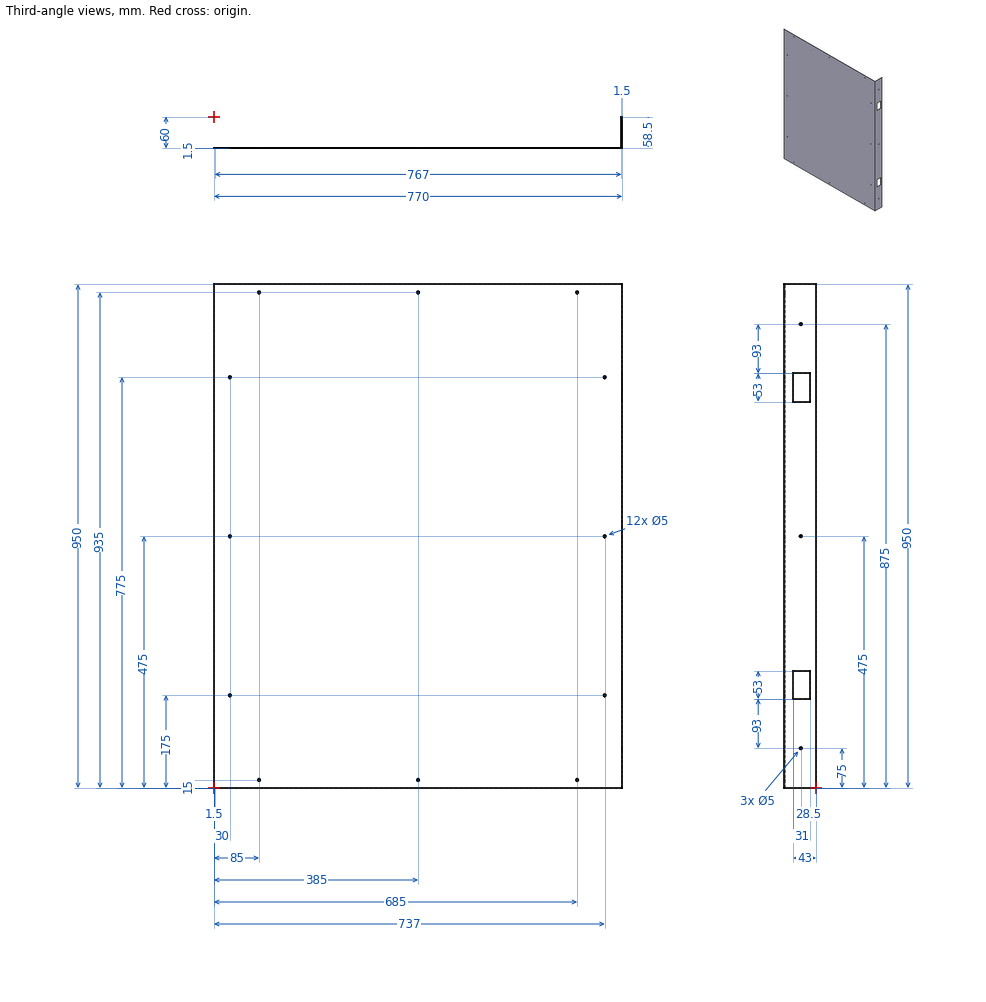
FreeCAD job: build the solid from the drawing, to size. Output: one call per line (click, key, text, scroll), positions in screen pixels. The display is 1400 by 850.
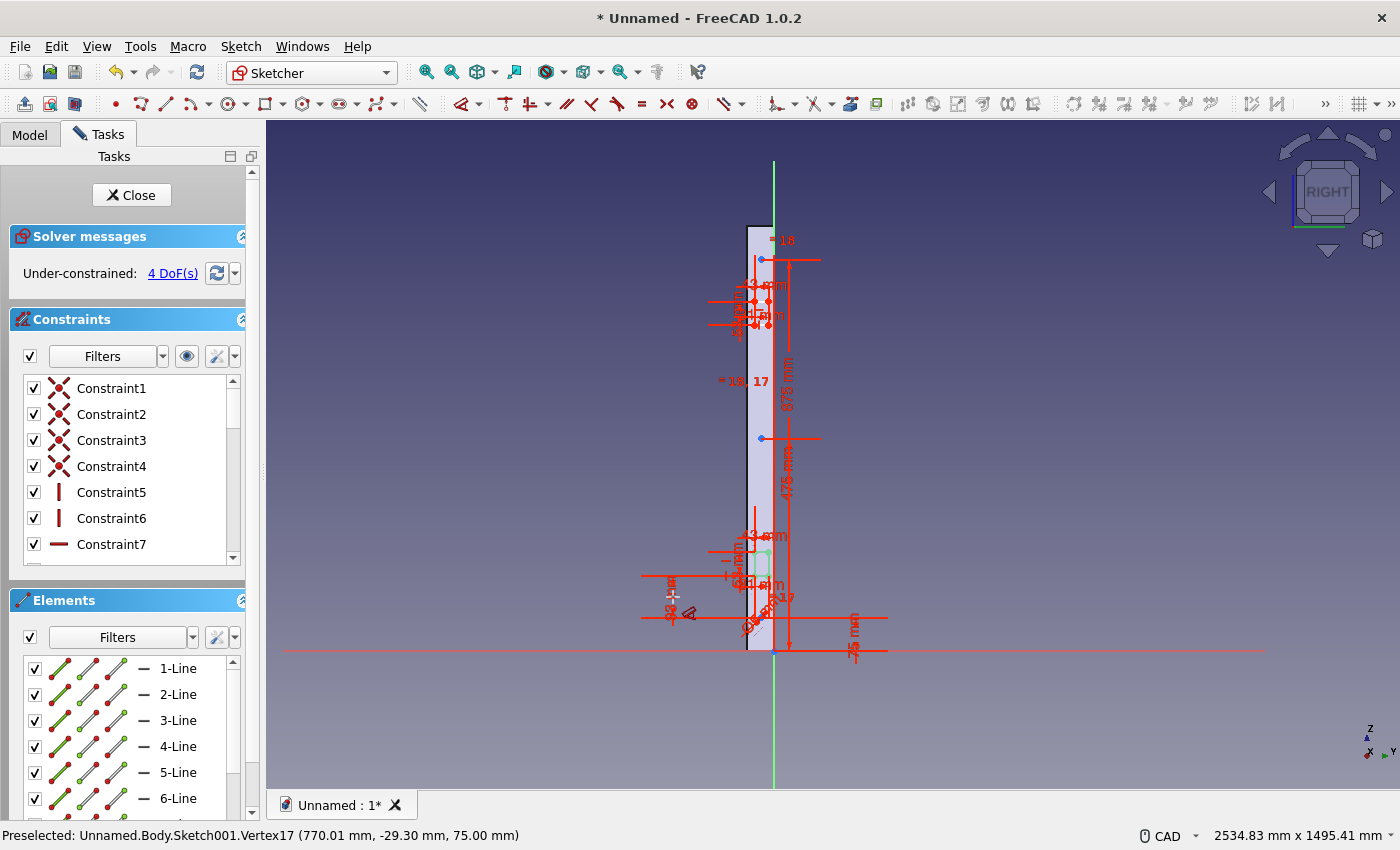
click(755, 302)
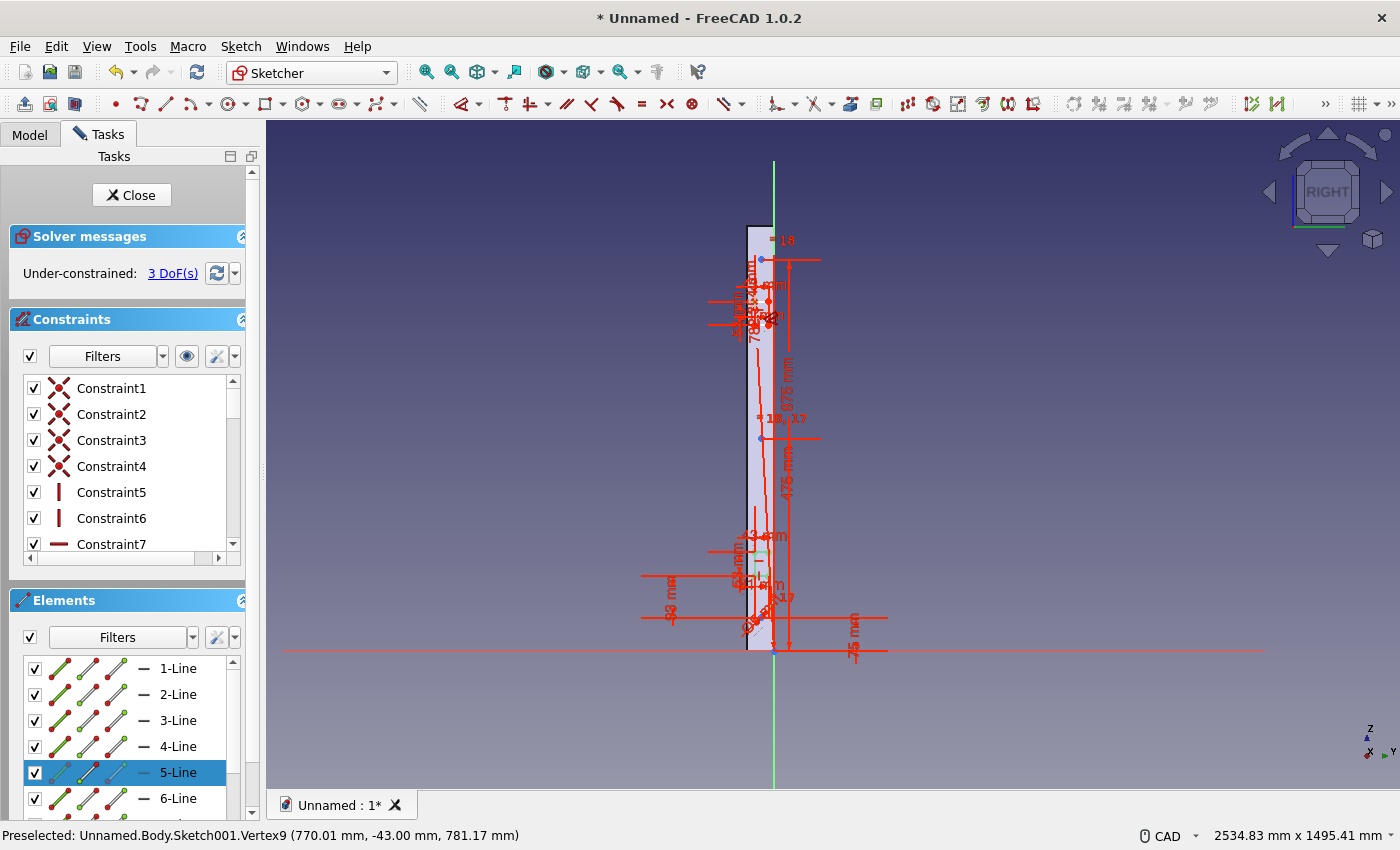
click(761, 260)
click(721, 266)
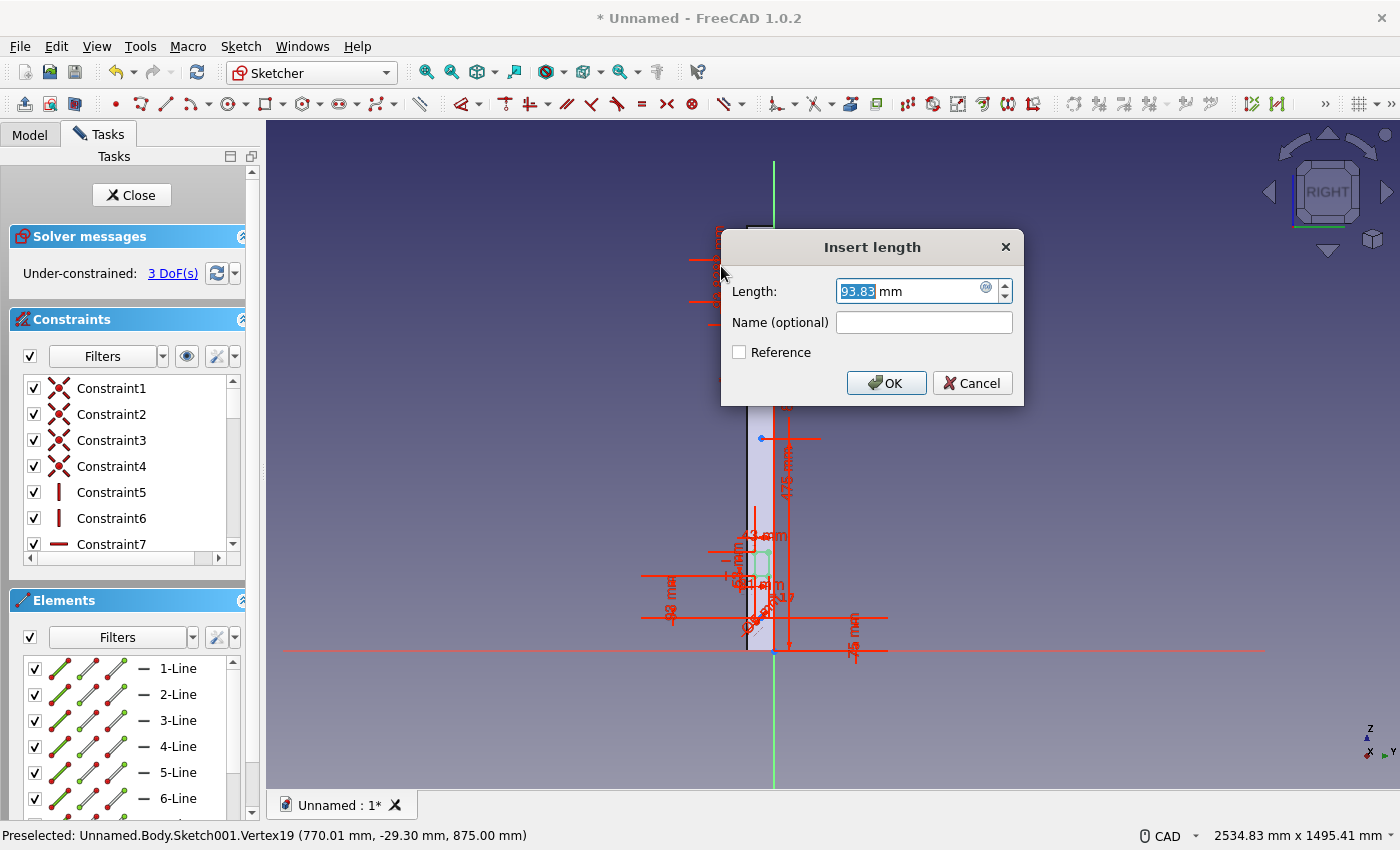
text(93)
key(Return)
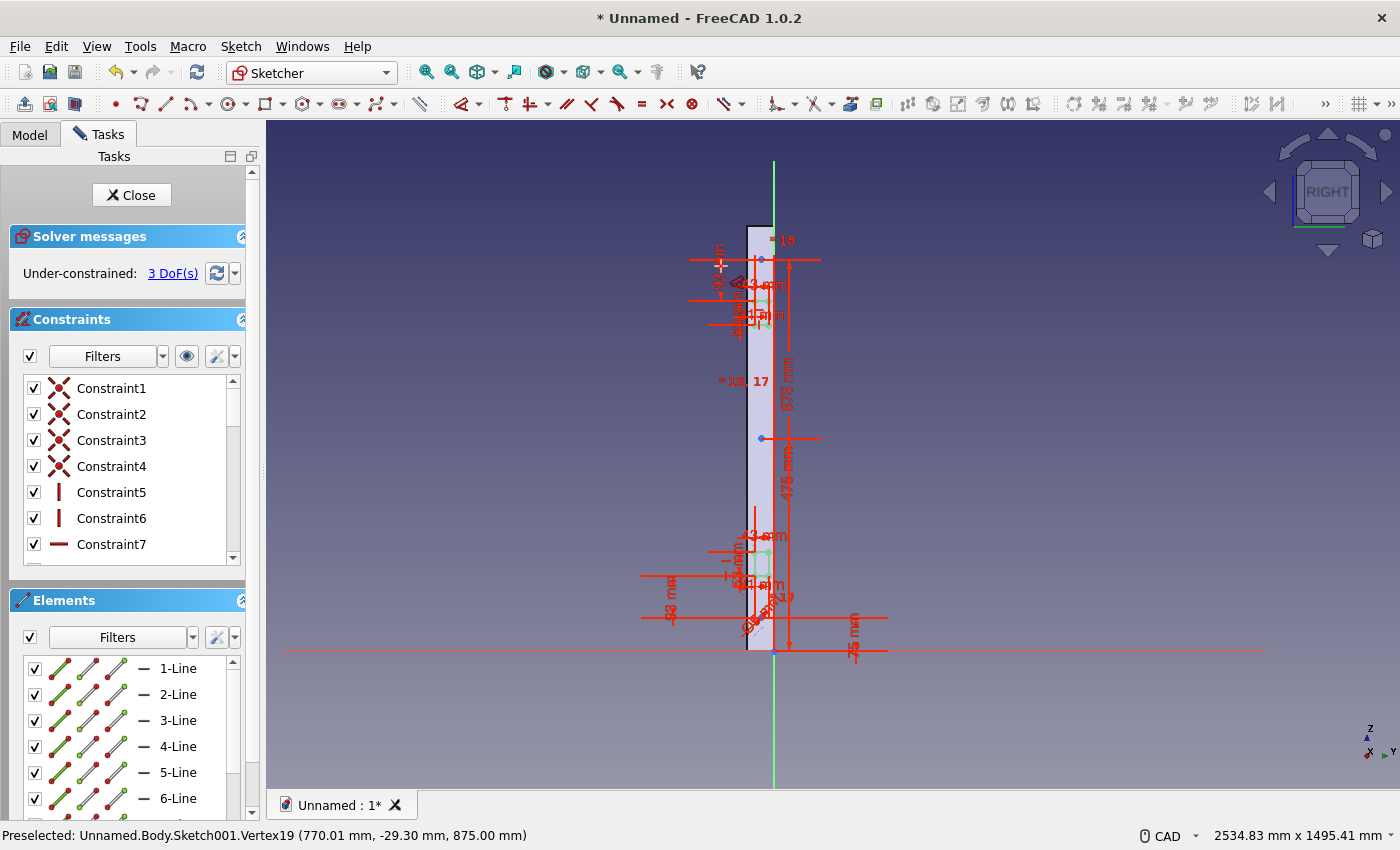
scroll(761, 618, up, 6)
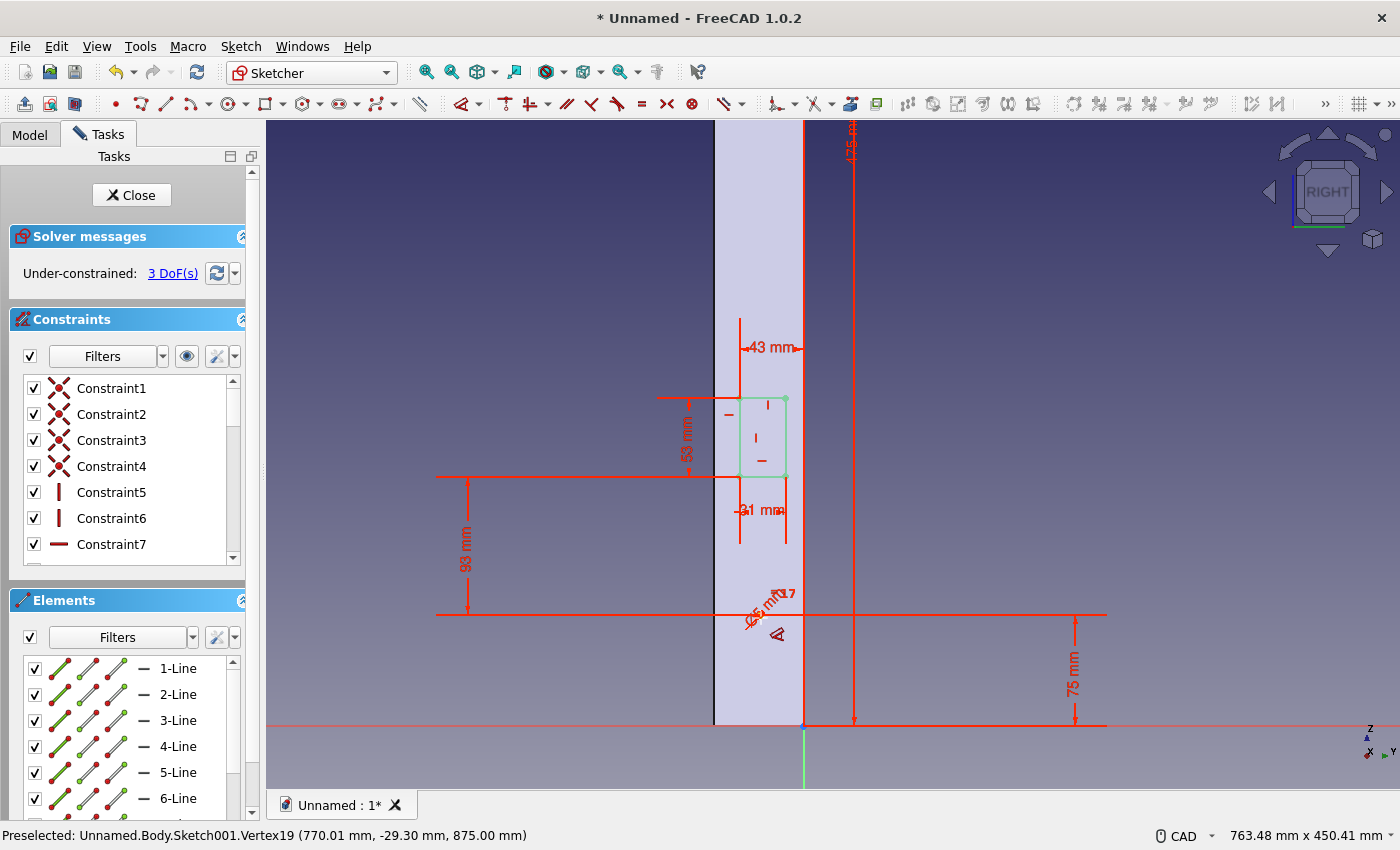
click(760, 615)
click(782, 760)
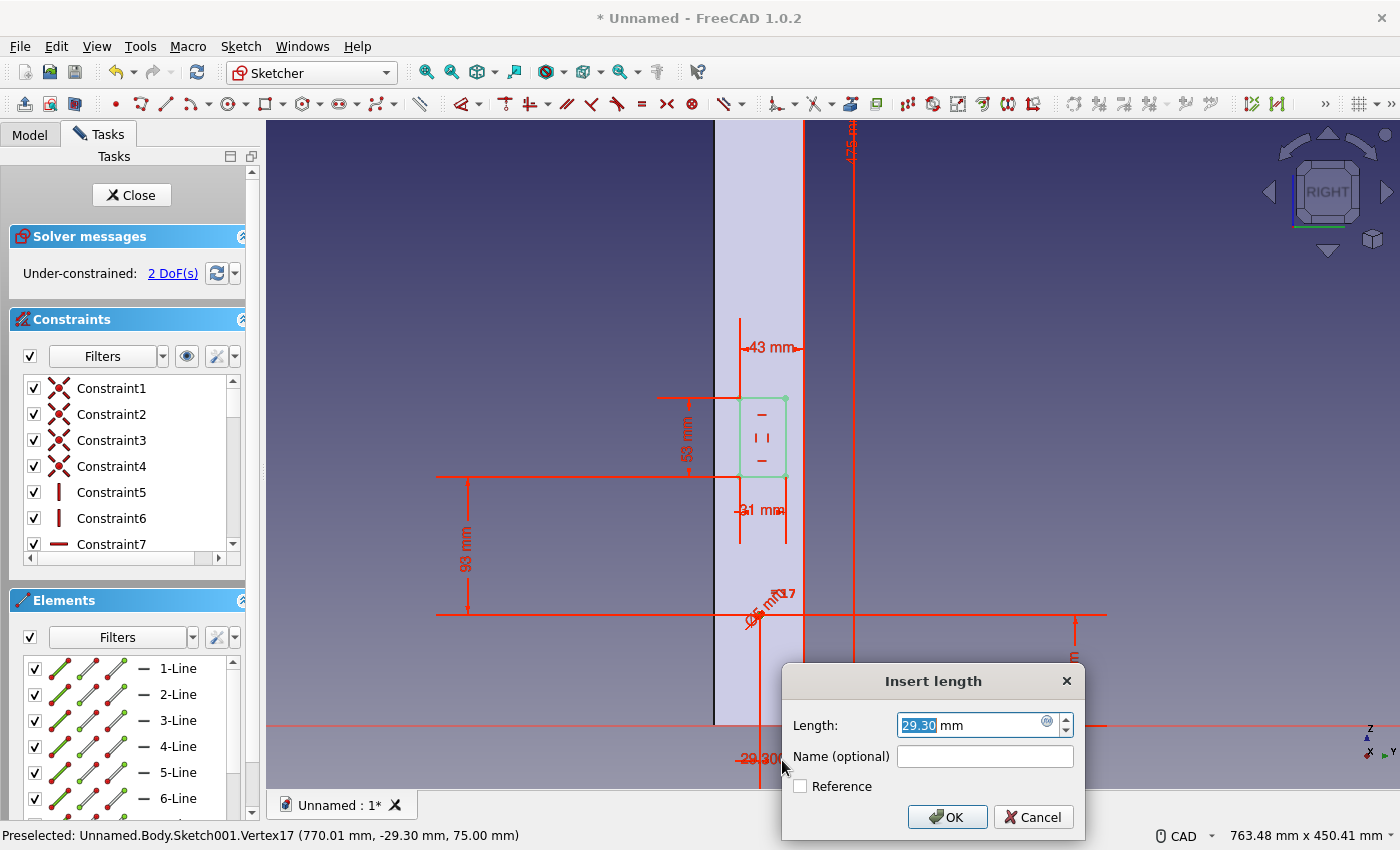
text(28.5)
key(Return)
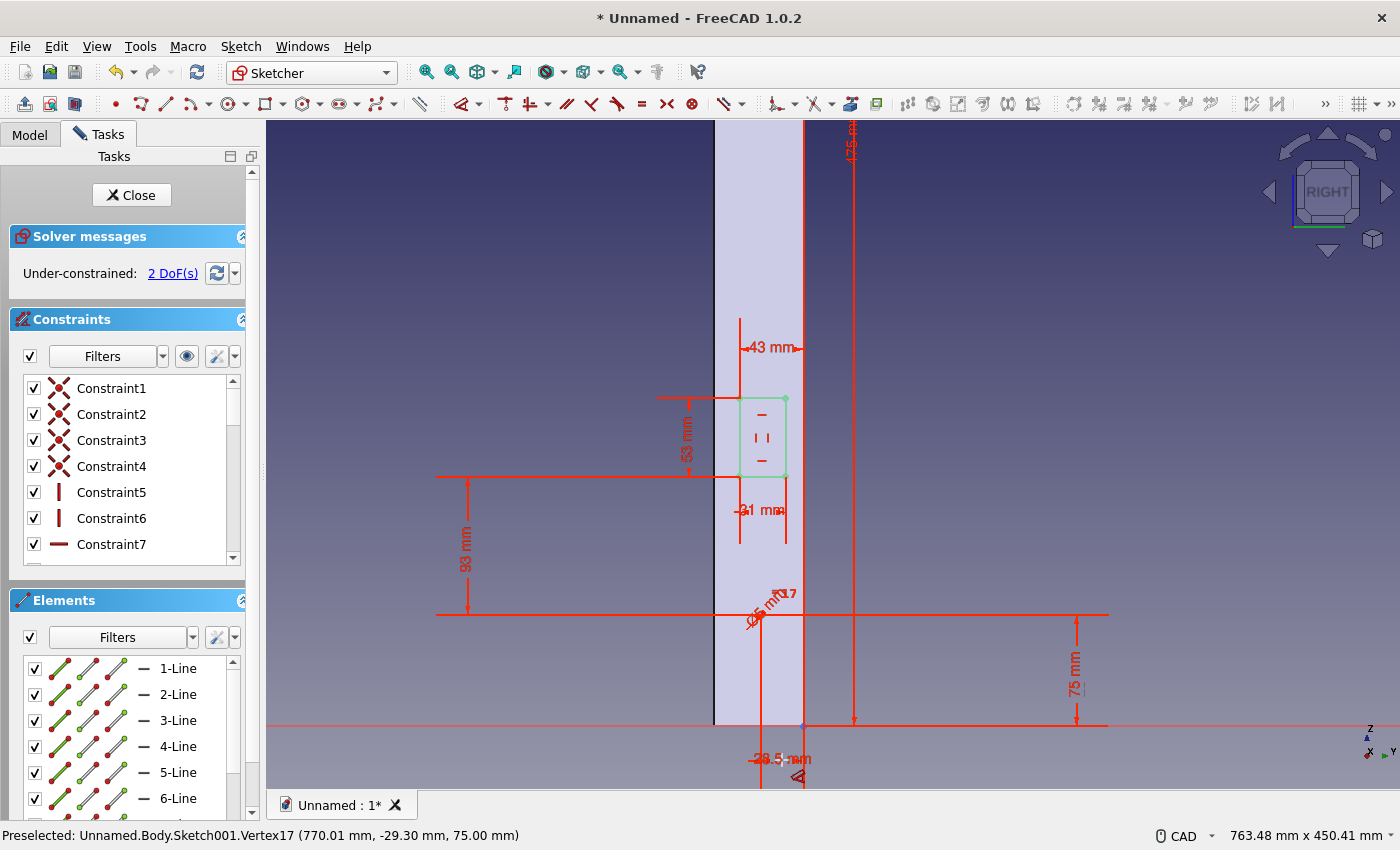
scroll(761, 618, down, 6)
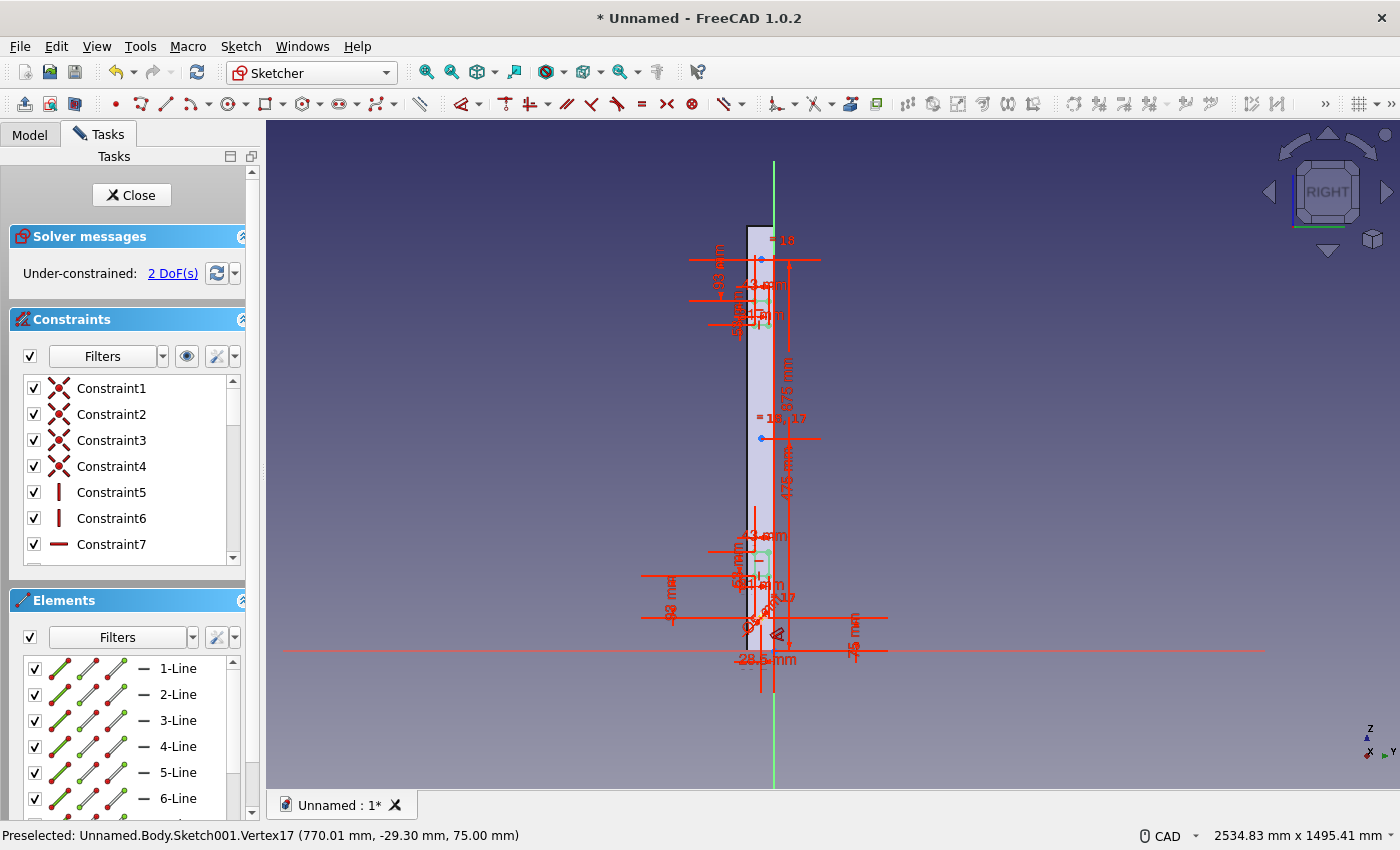
scroll(761, 439, up, 6)